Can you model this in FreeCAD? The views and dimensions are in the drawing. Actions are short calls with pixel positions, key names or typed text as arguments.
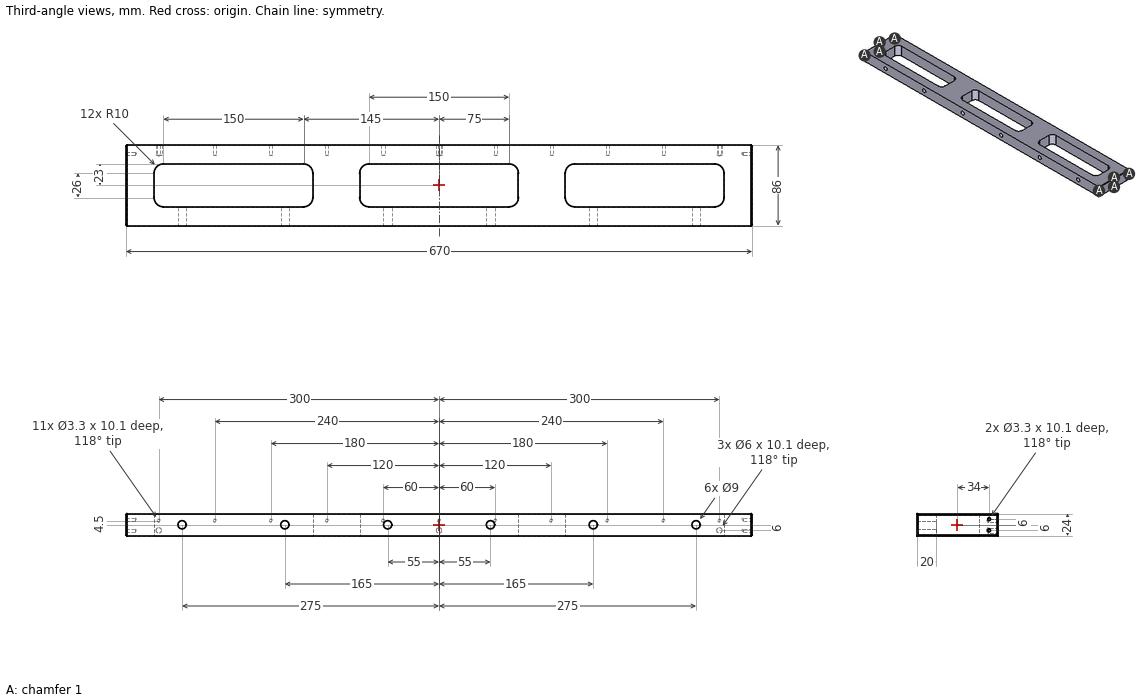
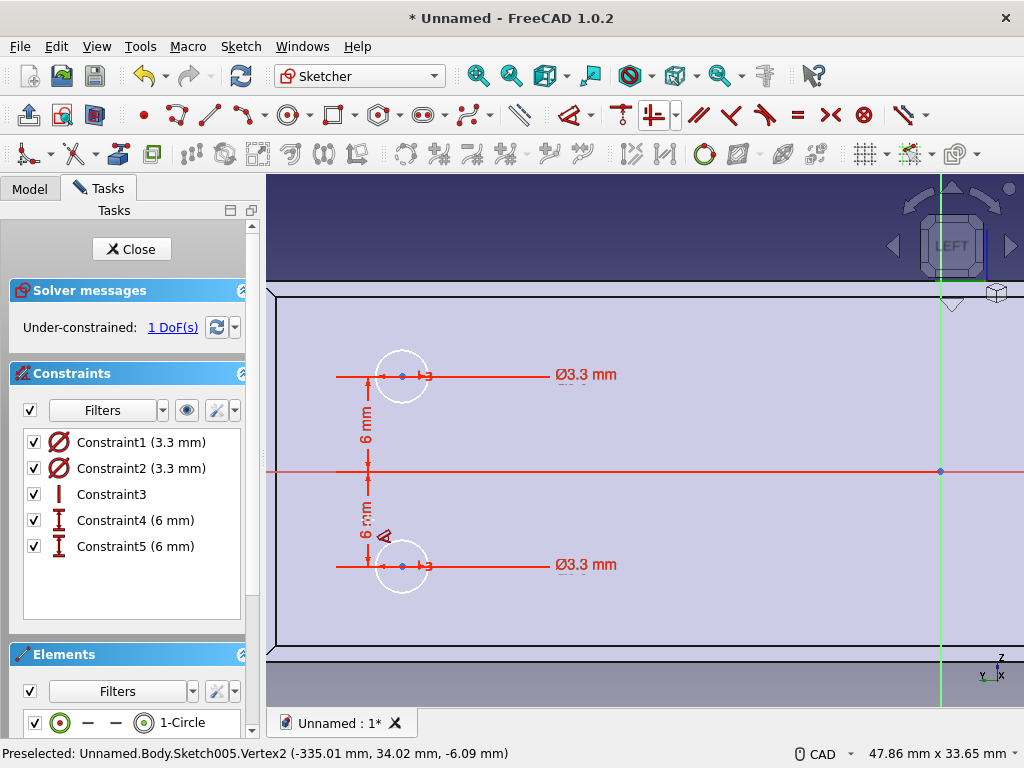
click(402, 377)
click(631, 343)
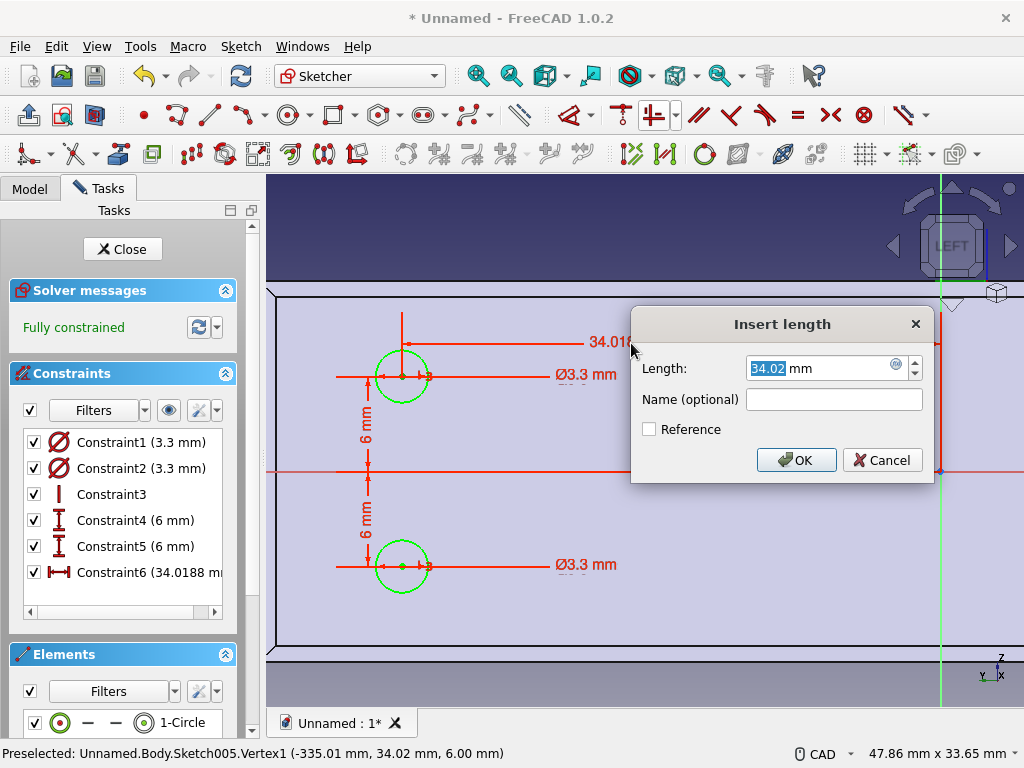
text(34)
key(Return)
key(Escape)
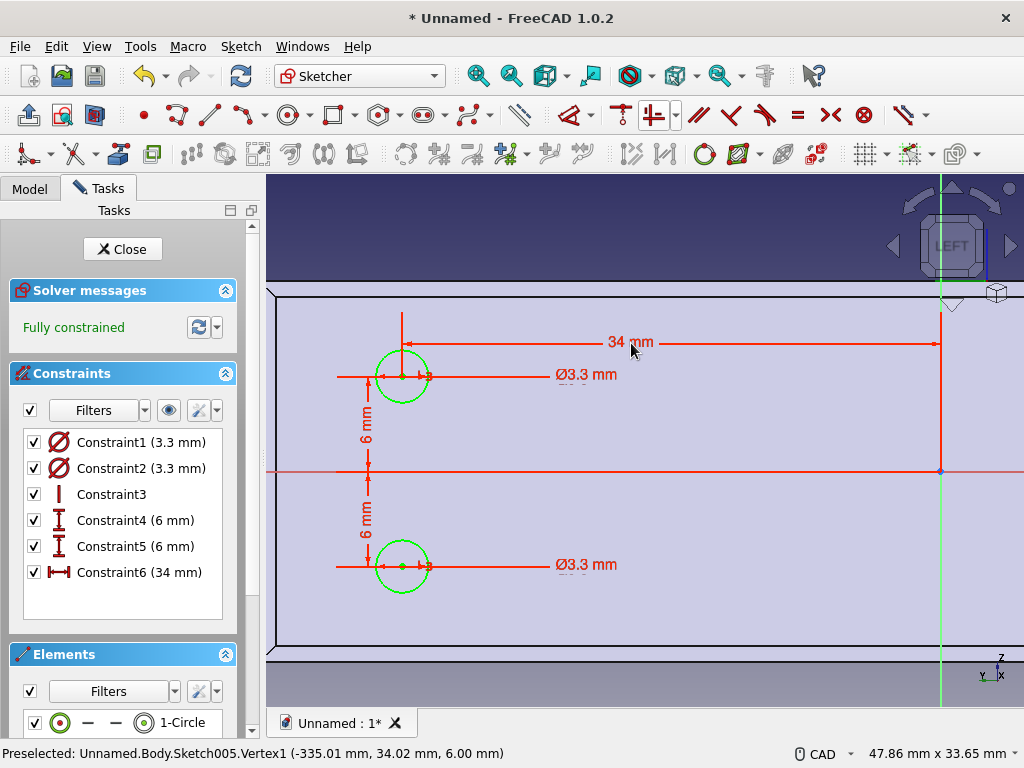
click(123, 249)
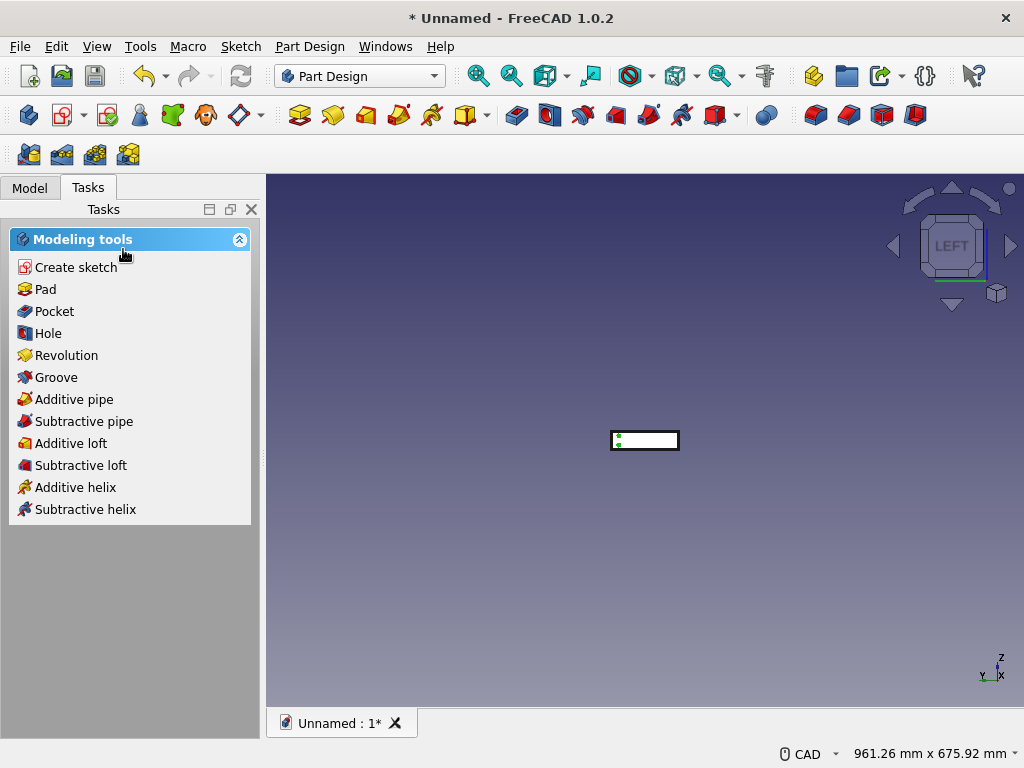
click(550, 116)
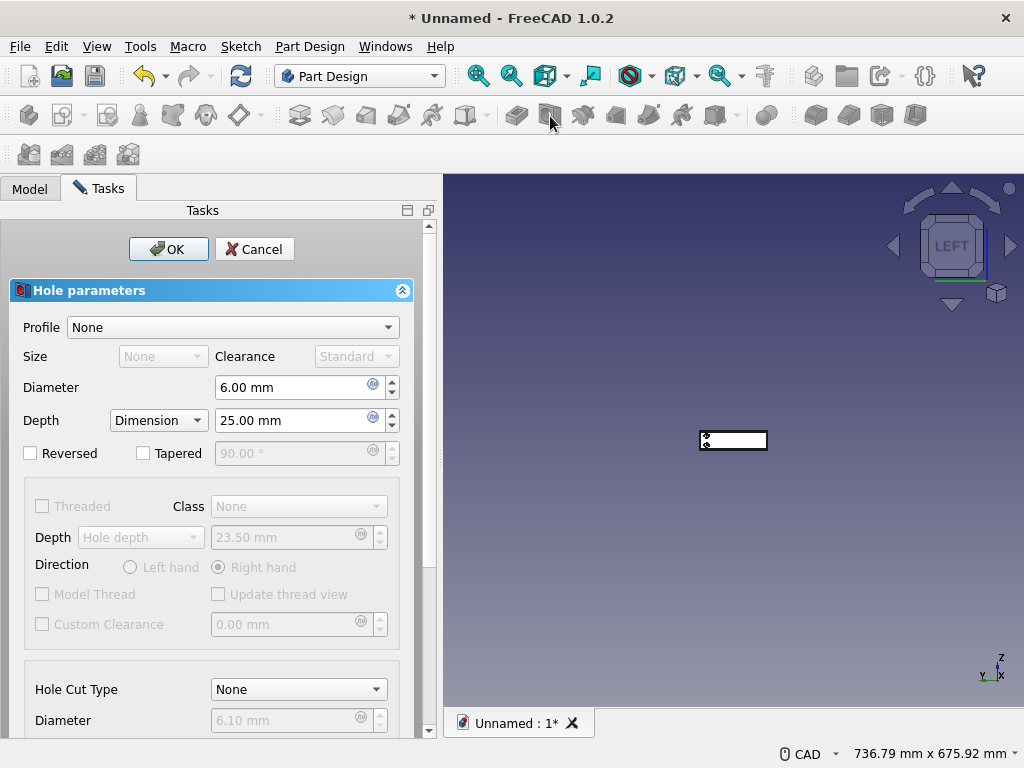
triple_click(300, 388)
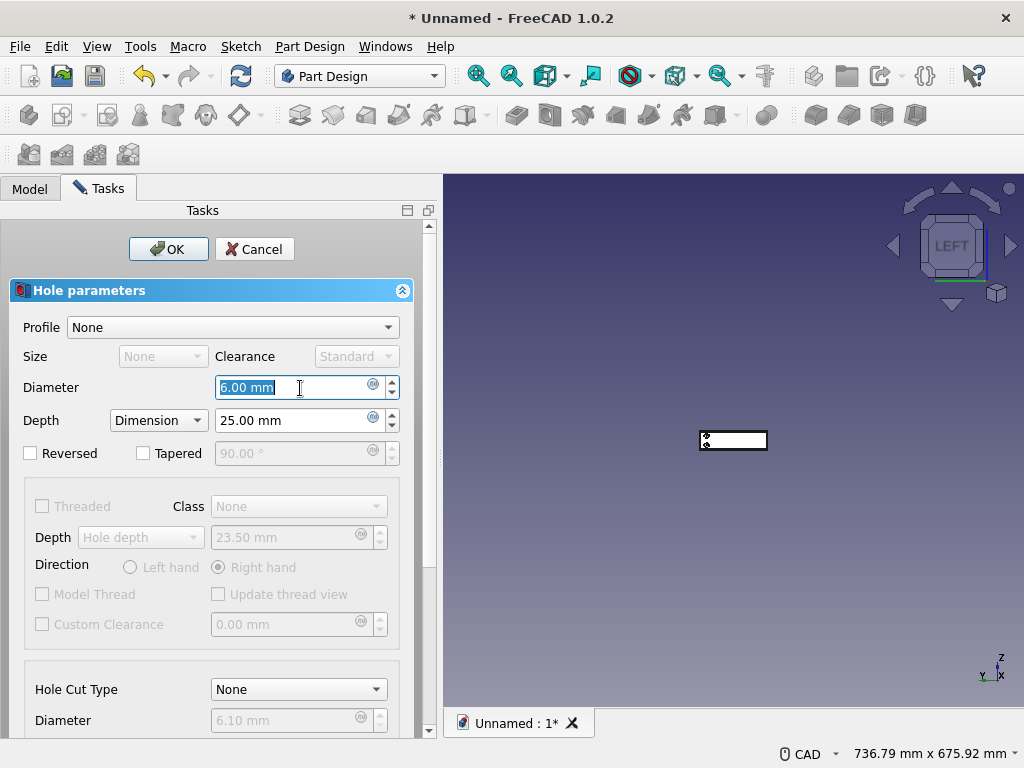
text(3.3)
key(Tab)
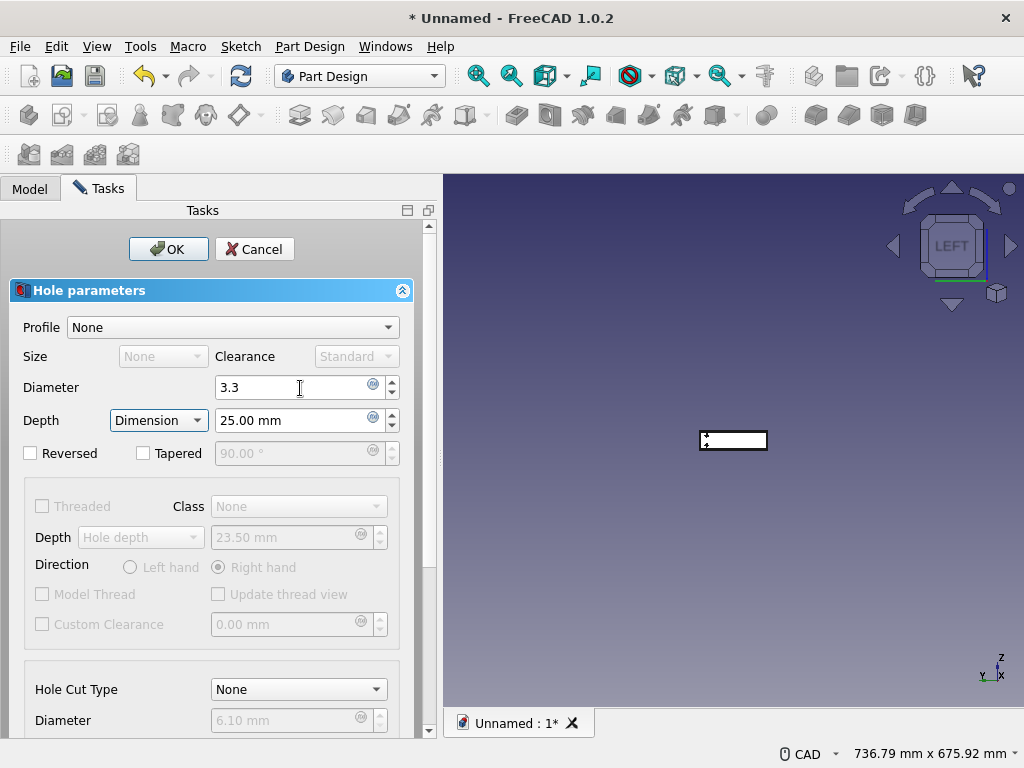
triple_click(300, 420)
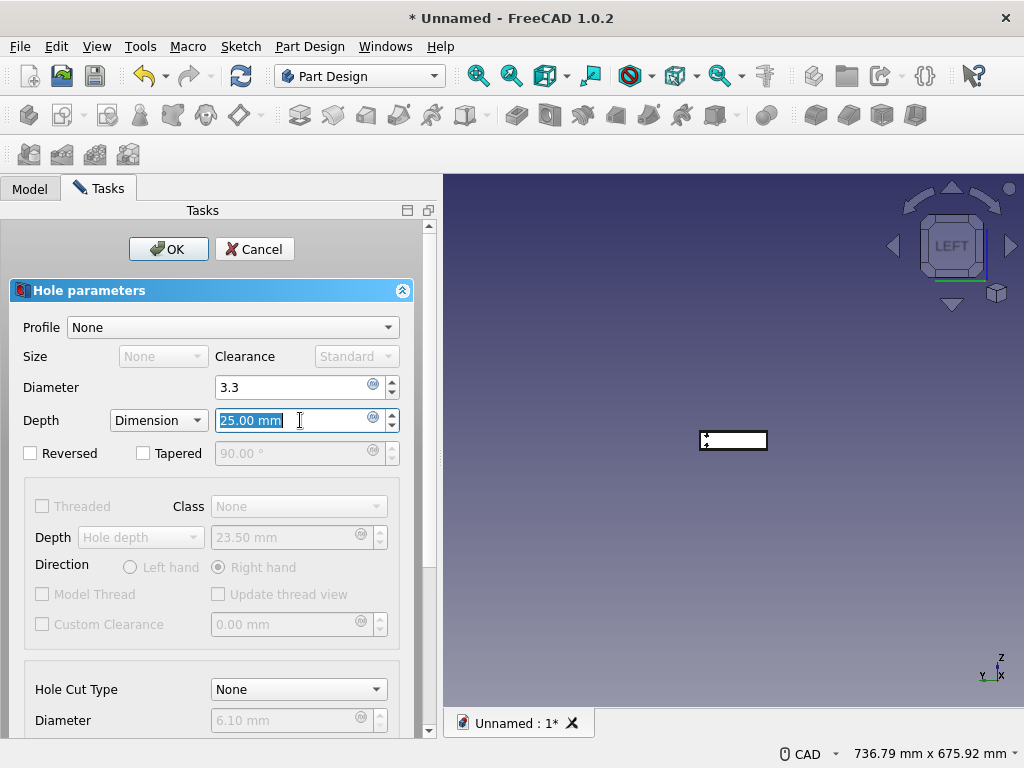
text(10.1)
key(Tab)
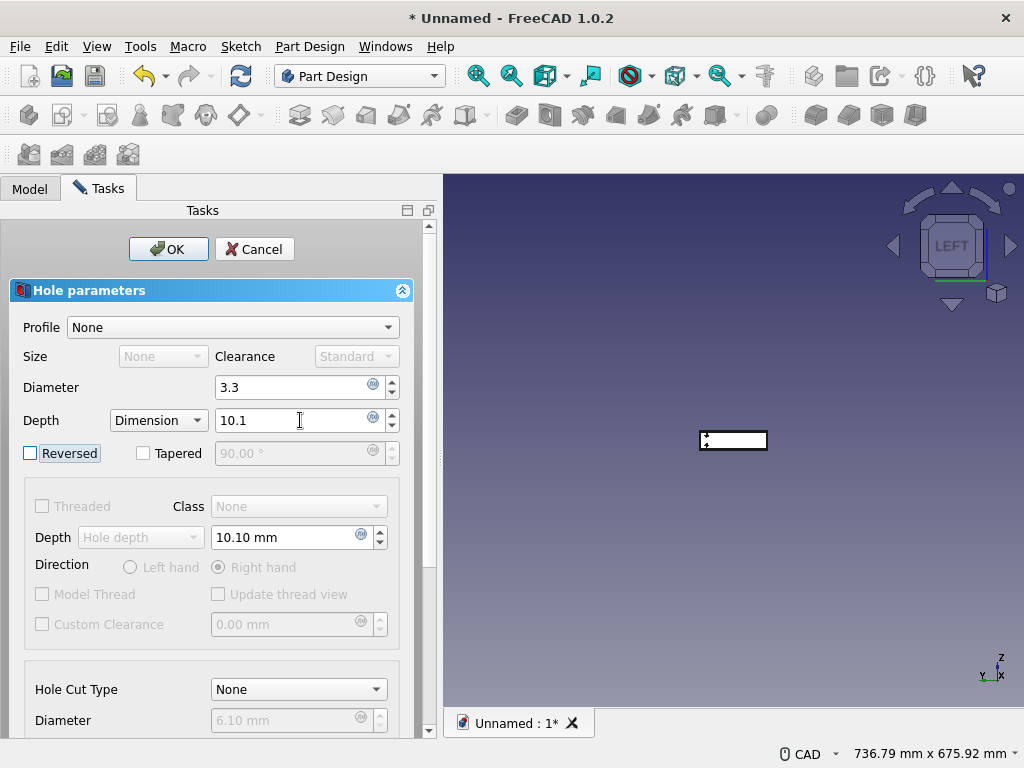
click(169, 249)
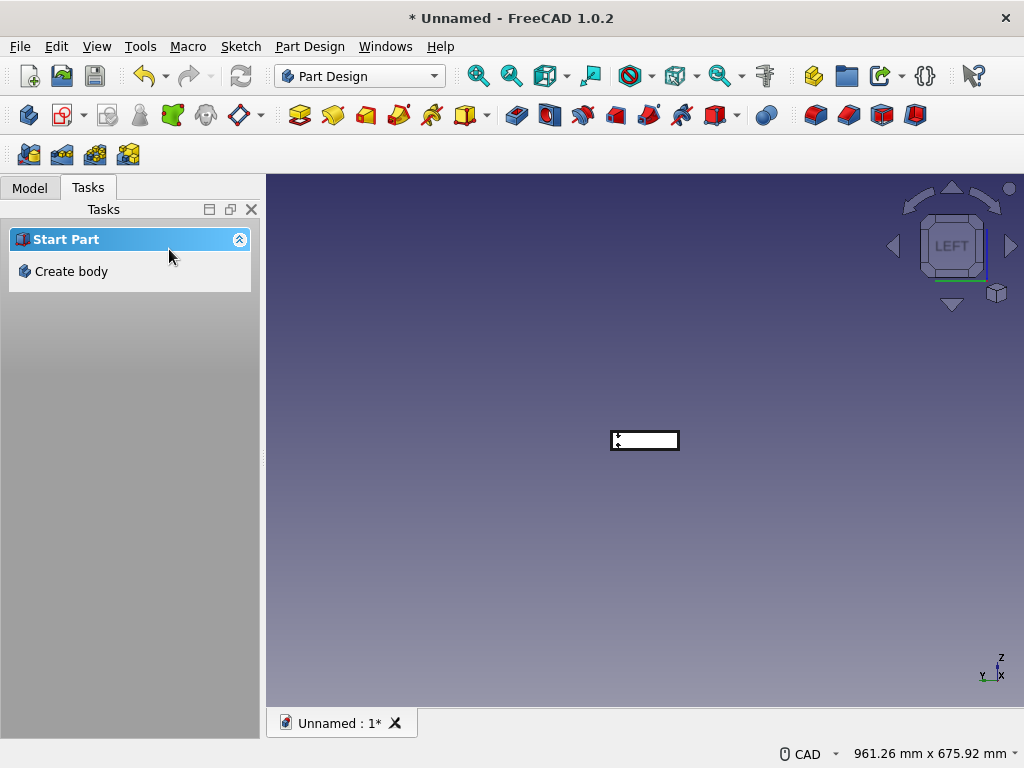
click(479, 76)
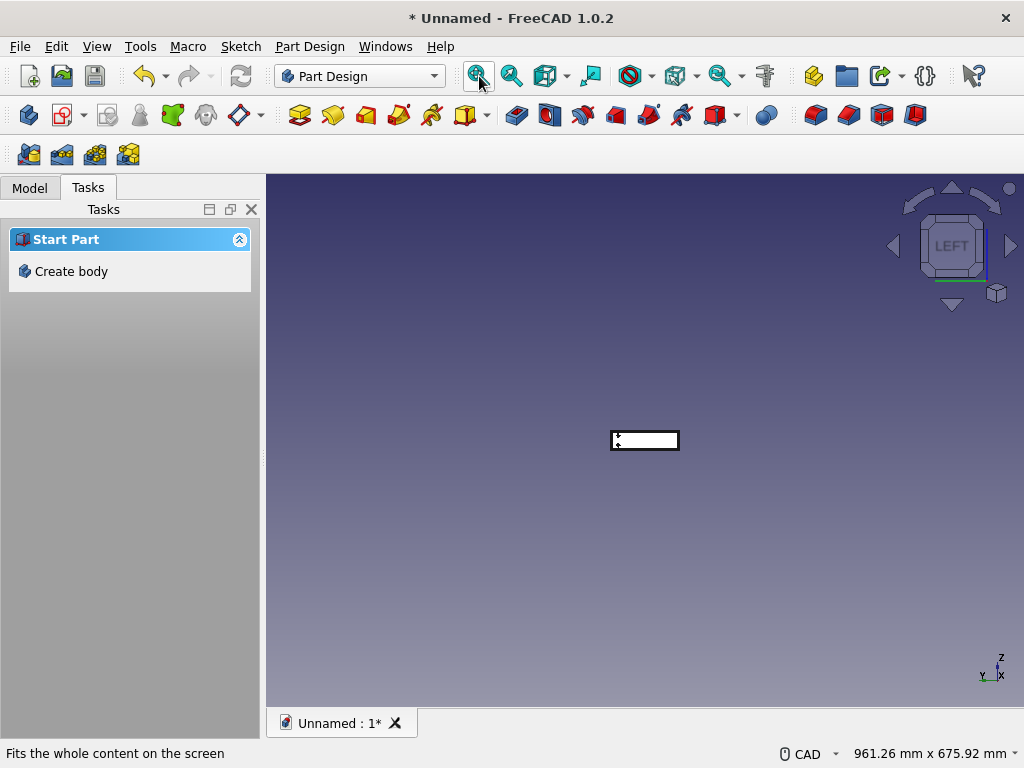
key(0)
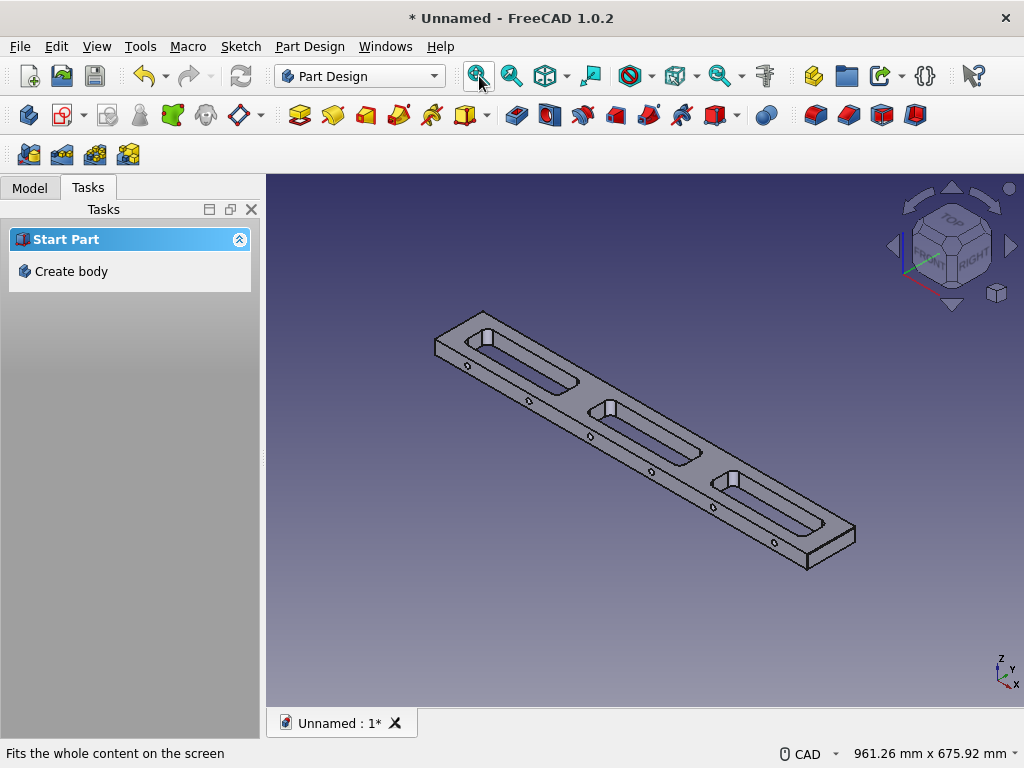
key(3)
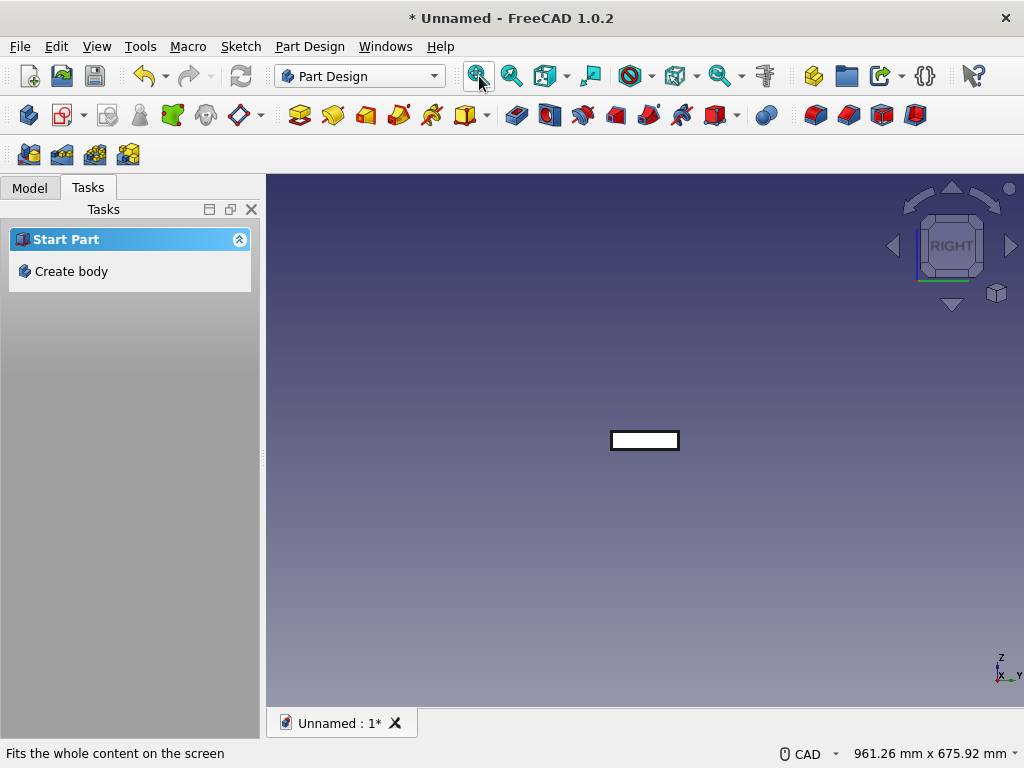
click(479, 76)